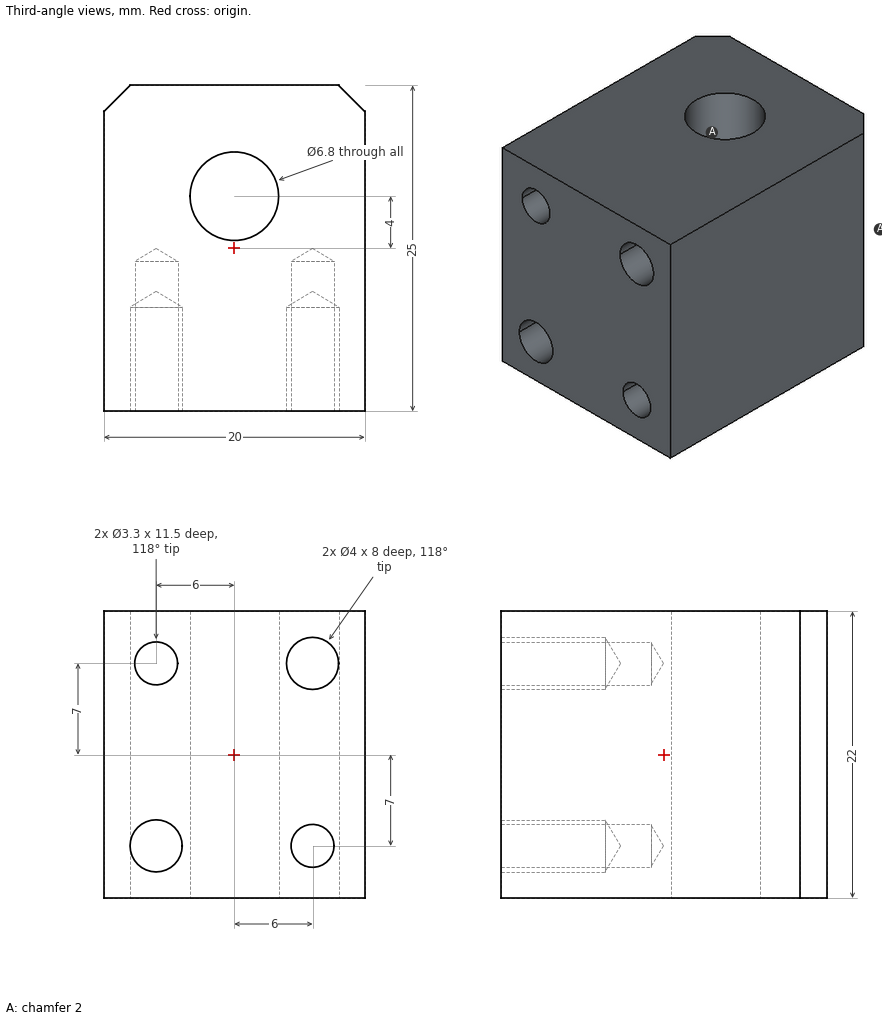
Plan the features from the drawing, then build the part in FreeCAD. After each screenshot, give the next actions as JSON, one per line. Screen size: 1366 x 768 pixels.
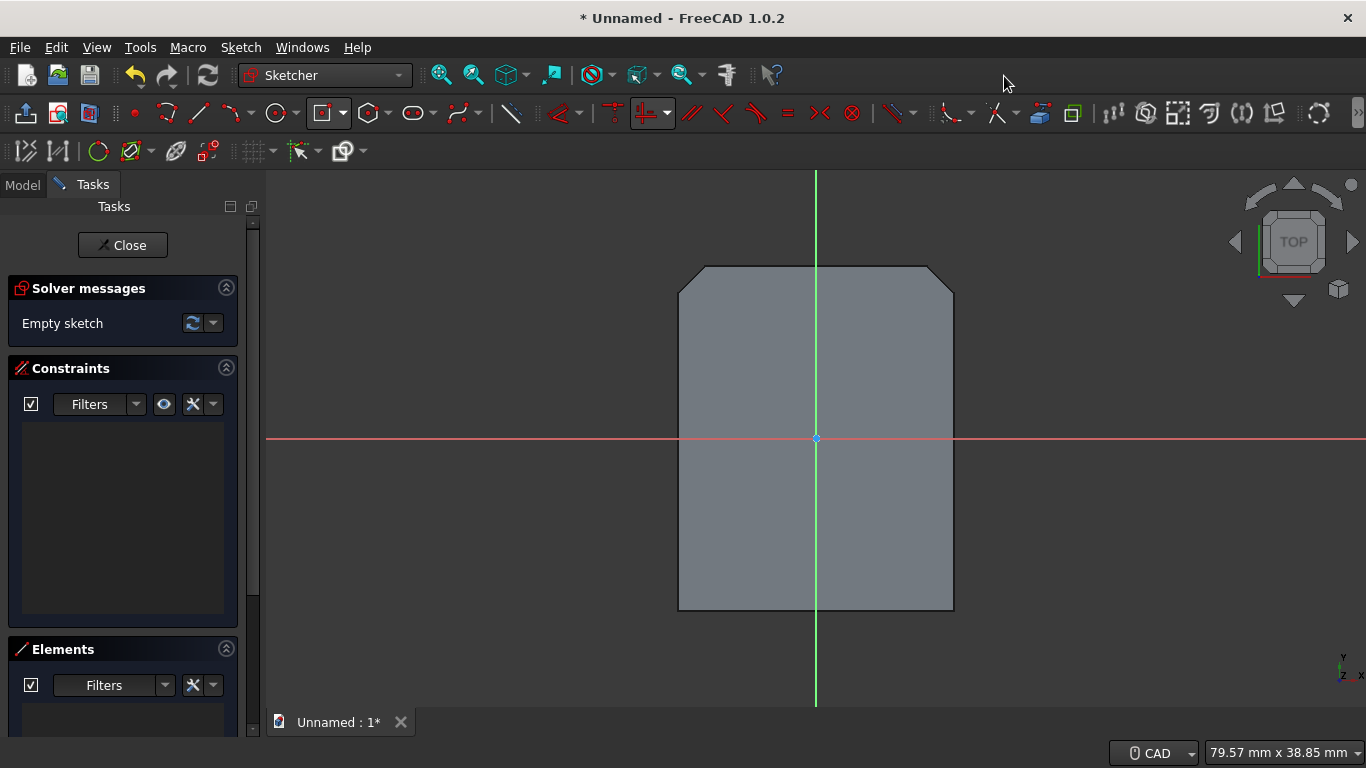
{"action": "scroll", "coordinate": [846, 365], "scroll_direction": "up", "scroll_amount": 6}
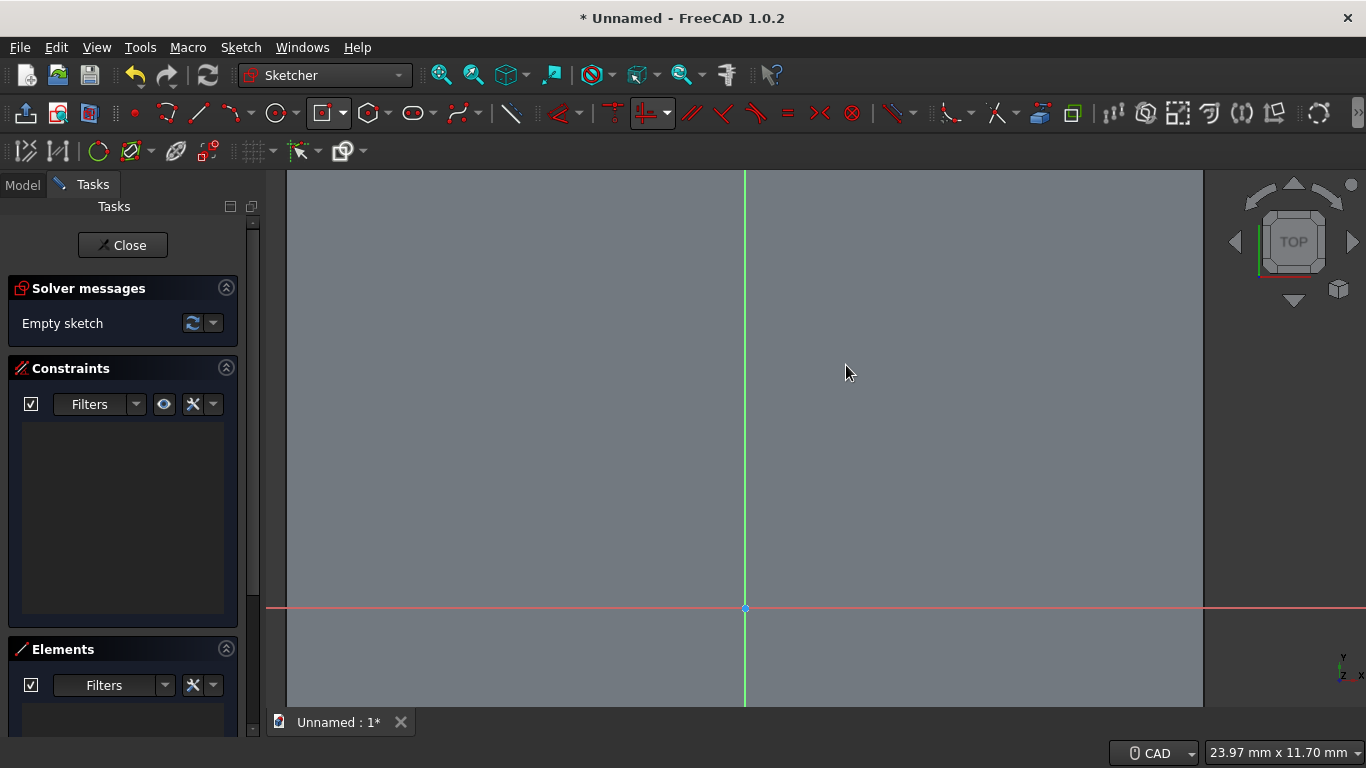
{"action": "left_click", "coordinate": [276, 114]}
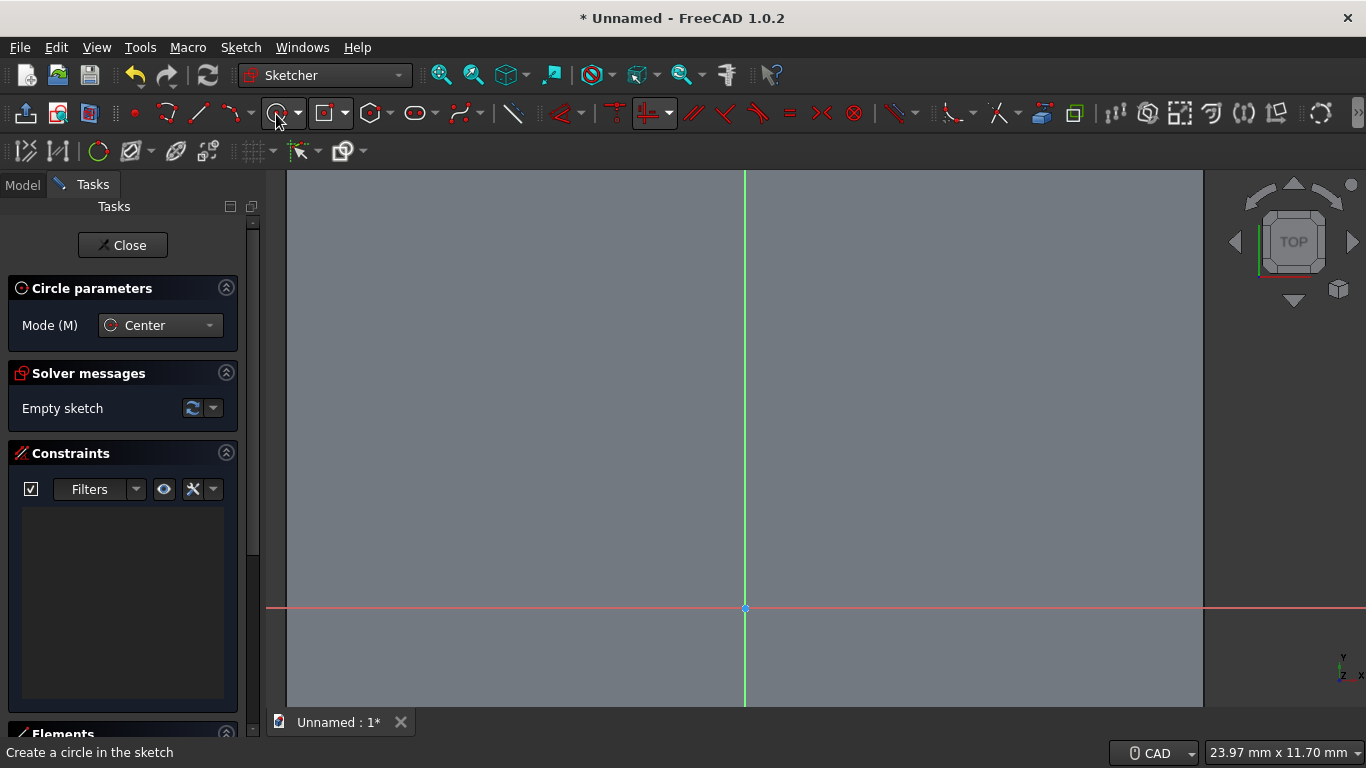
{"action": "left_click", "coordinate": [745, 425]}
{"action": "mouse_move", "coordinate": [856, 314]}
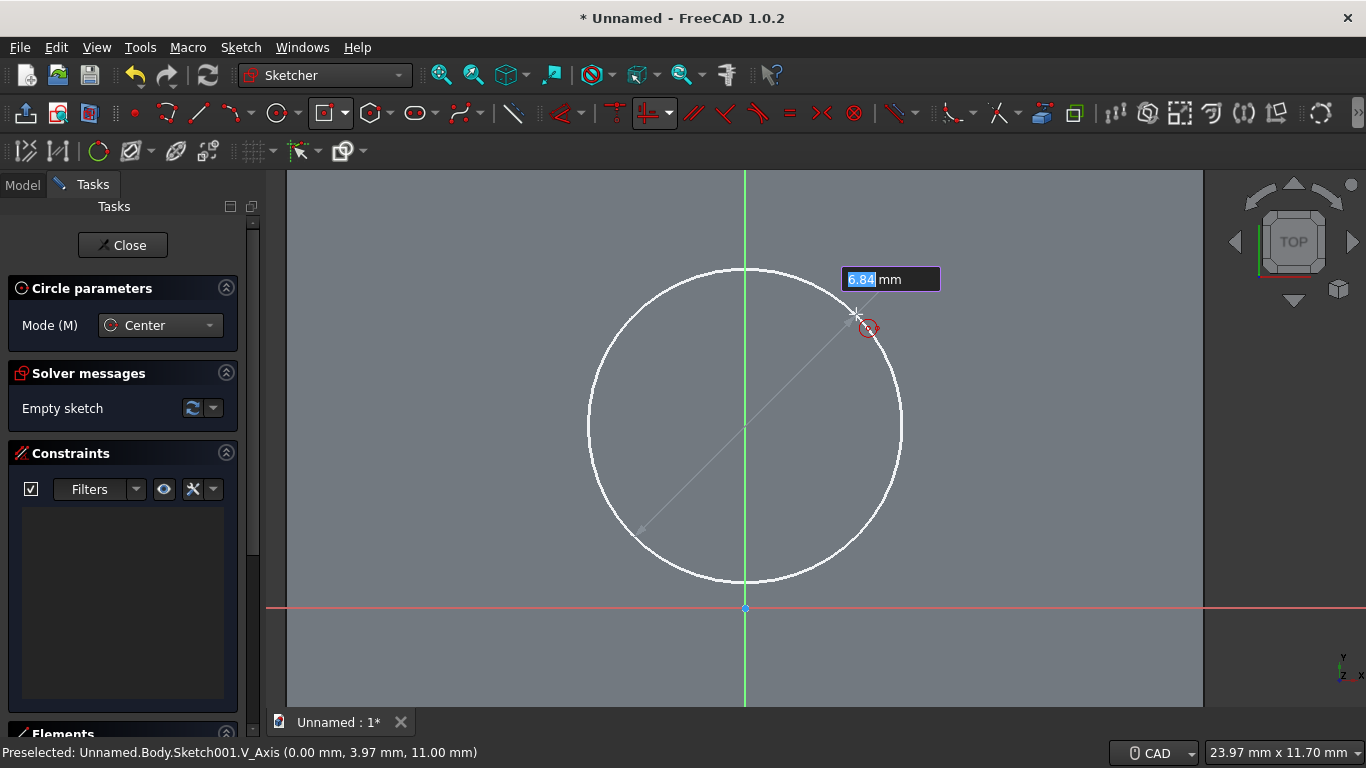
{"action": "type", "text": "6.8"}
{"action": "key", "text": "Return"}
{"action": "key", "text": "Escape"}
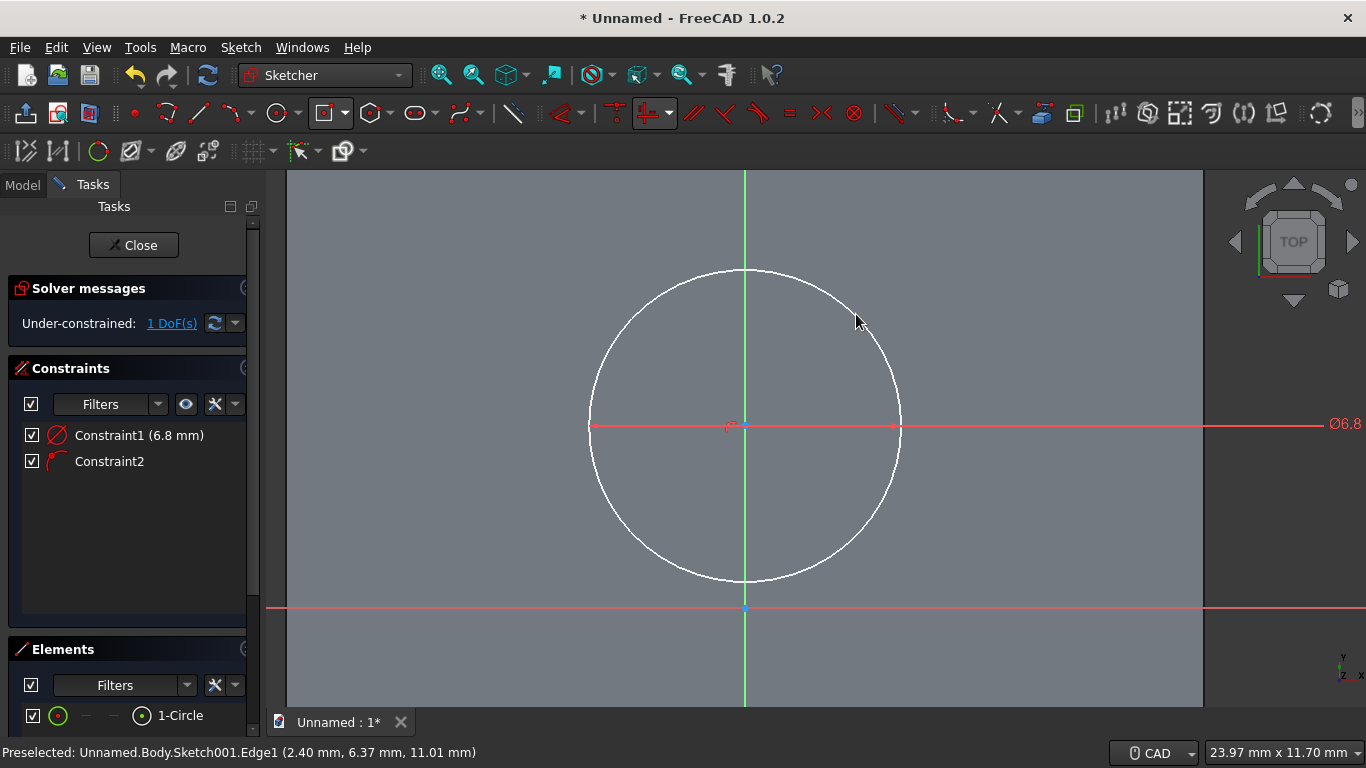
{"action": "left_click", "coordinate": [745, 426]}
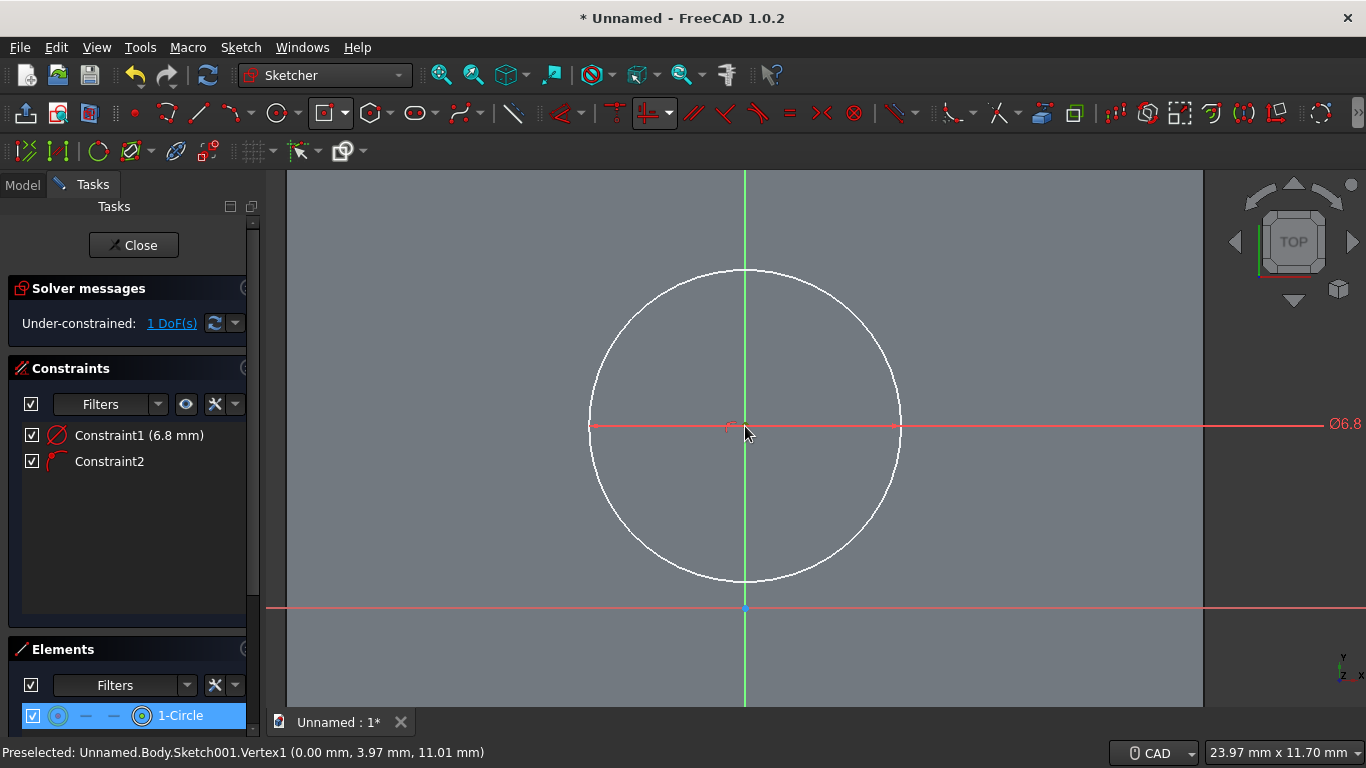
{"action": "key", "text": "i"}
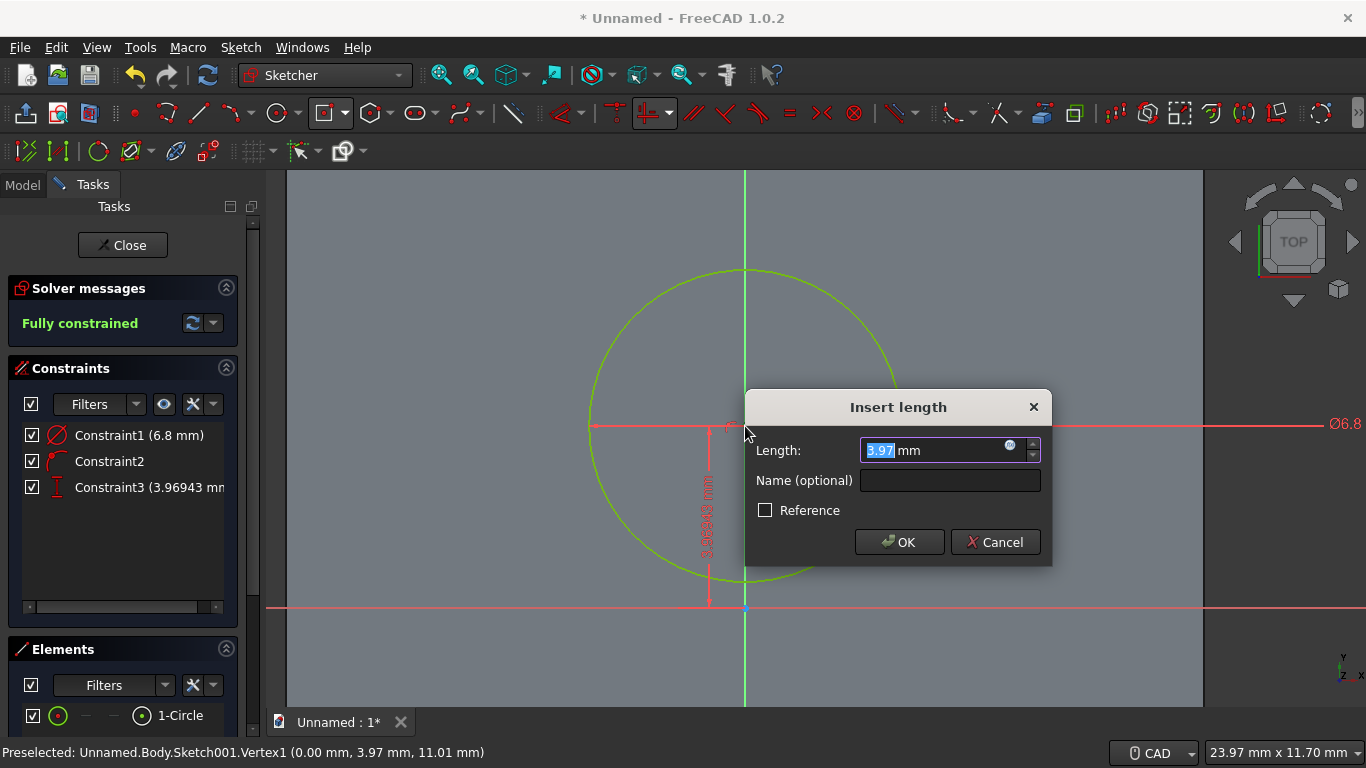
{"action": "type", "text": "4"}
{"action": "key", "text": "Return"}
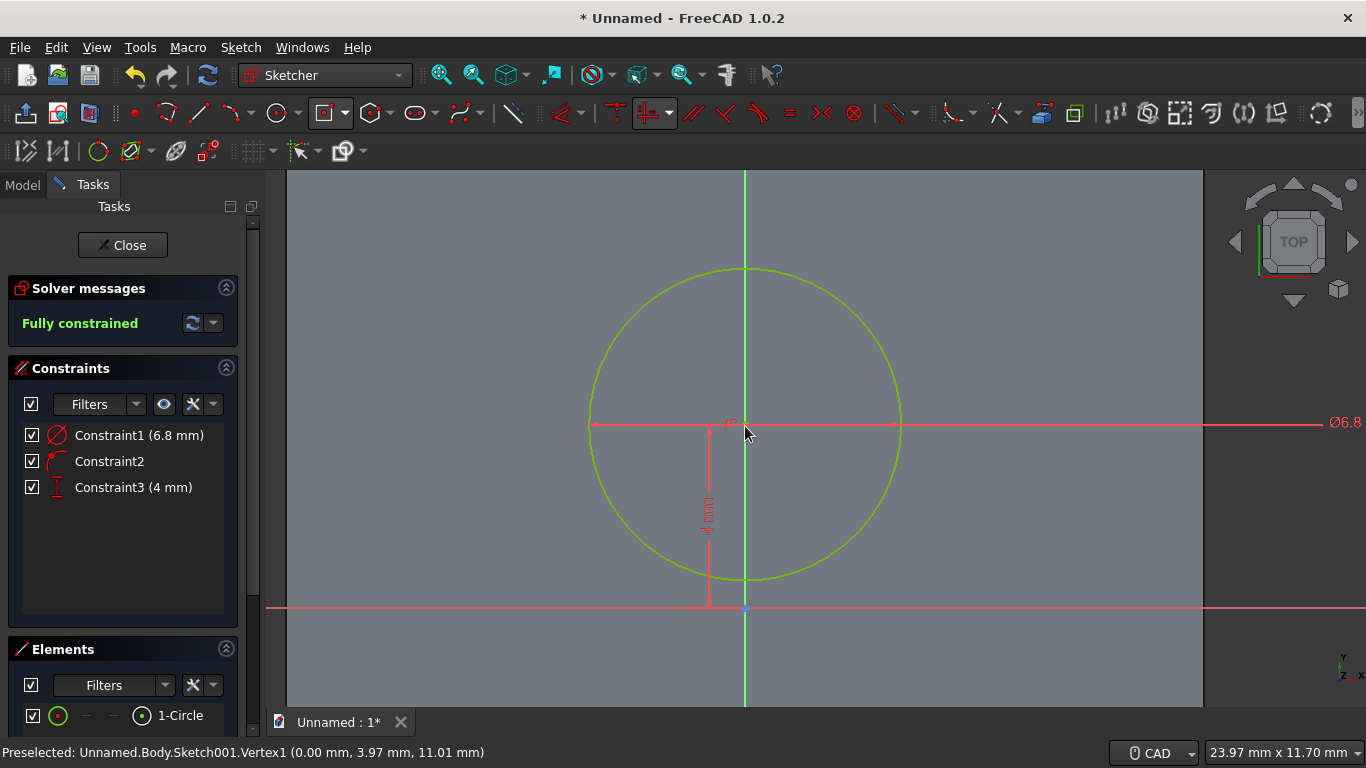
{"action": "left_click", "coordinate": [123, 245]}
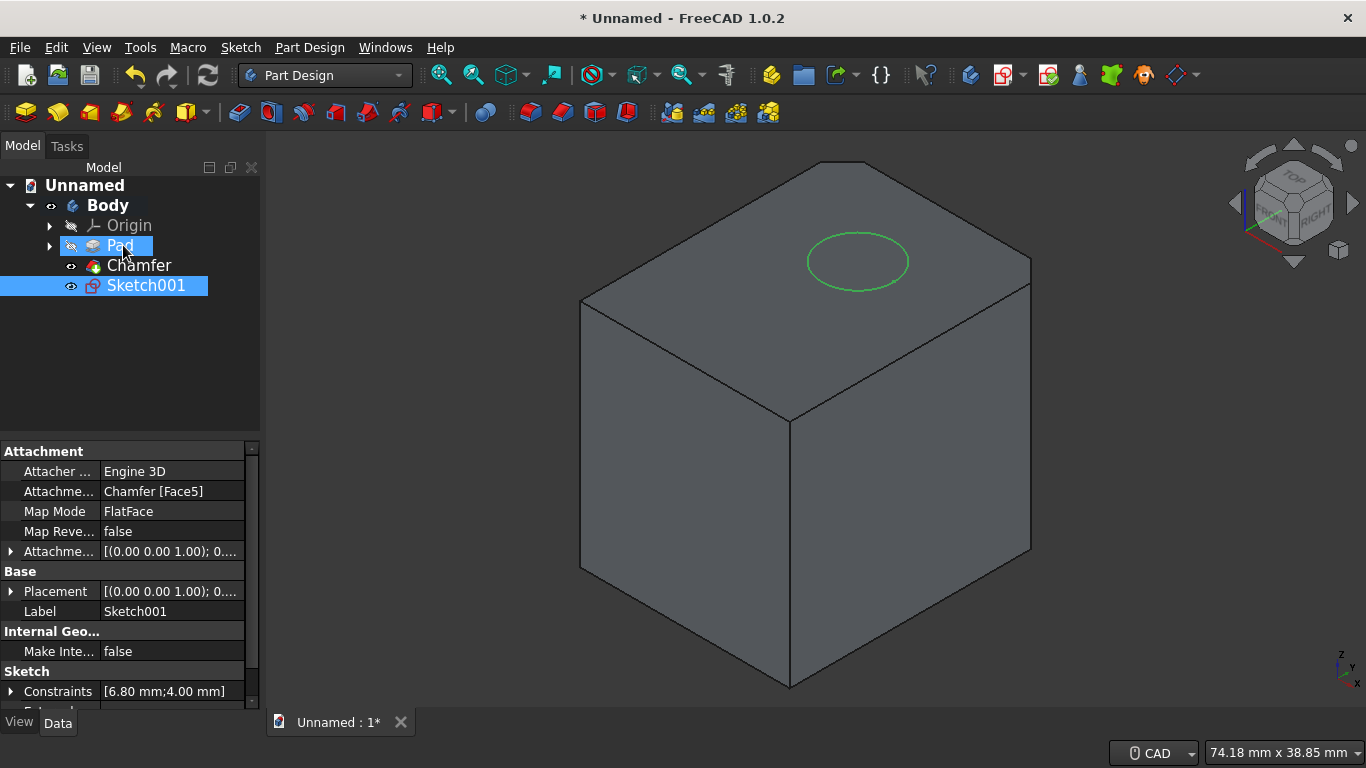
{"action": "left_click", "coordinate": [272, 112]}